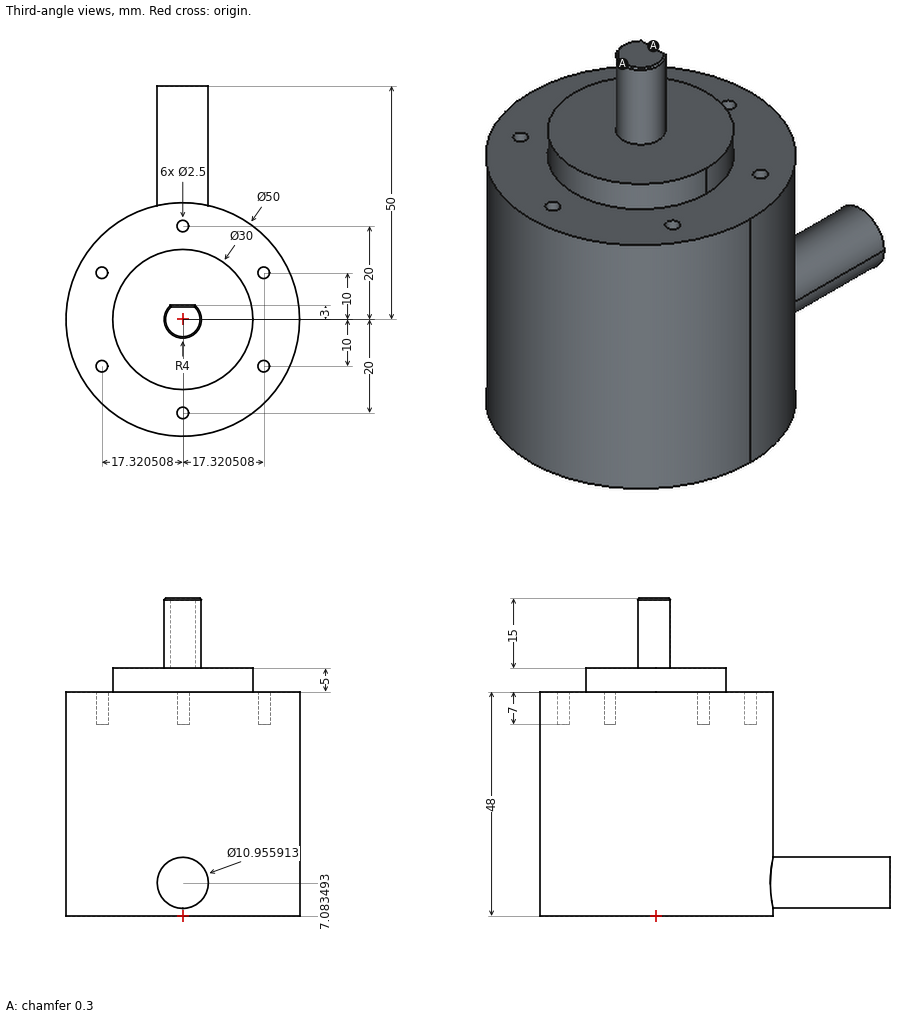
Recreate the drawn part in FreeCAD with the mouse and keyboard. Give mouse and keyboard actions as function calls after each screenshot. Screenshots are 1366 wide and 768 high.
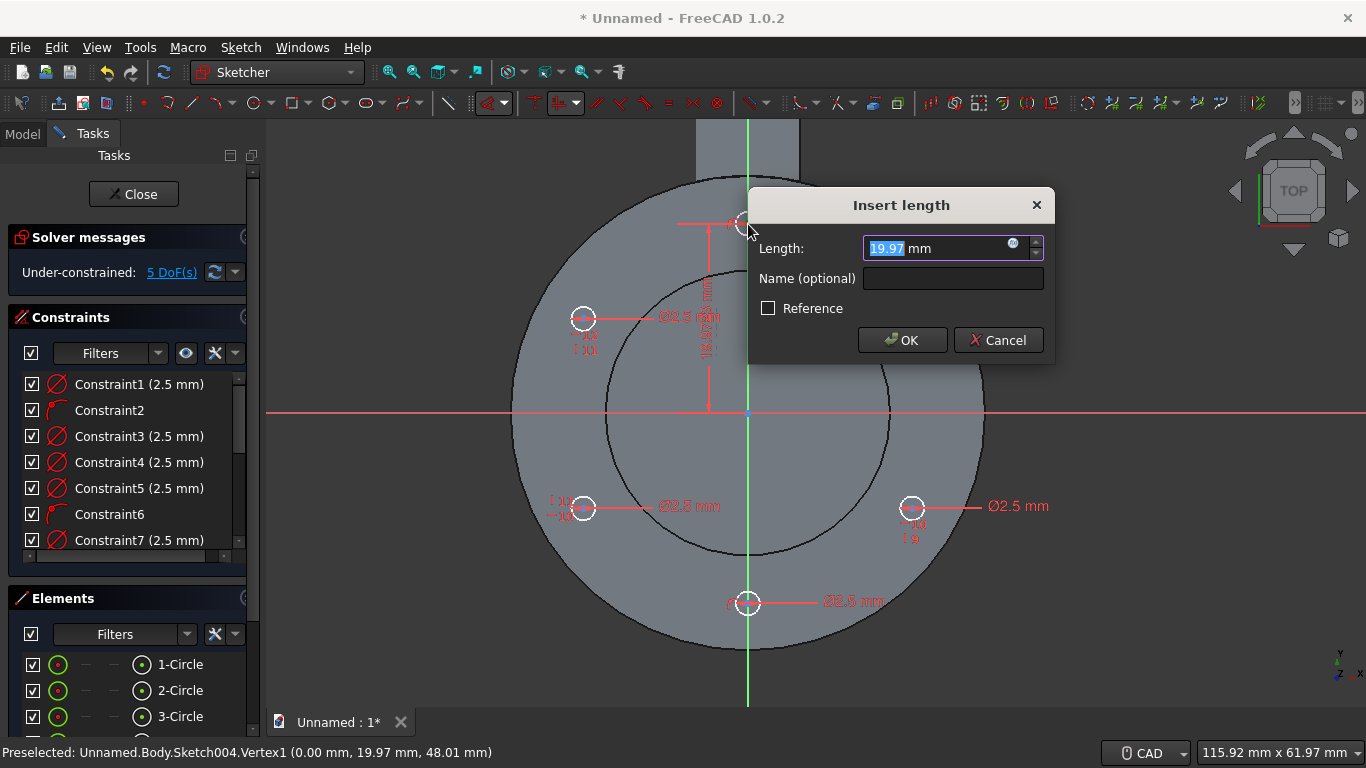
text(20)
key(Return)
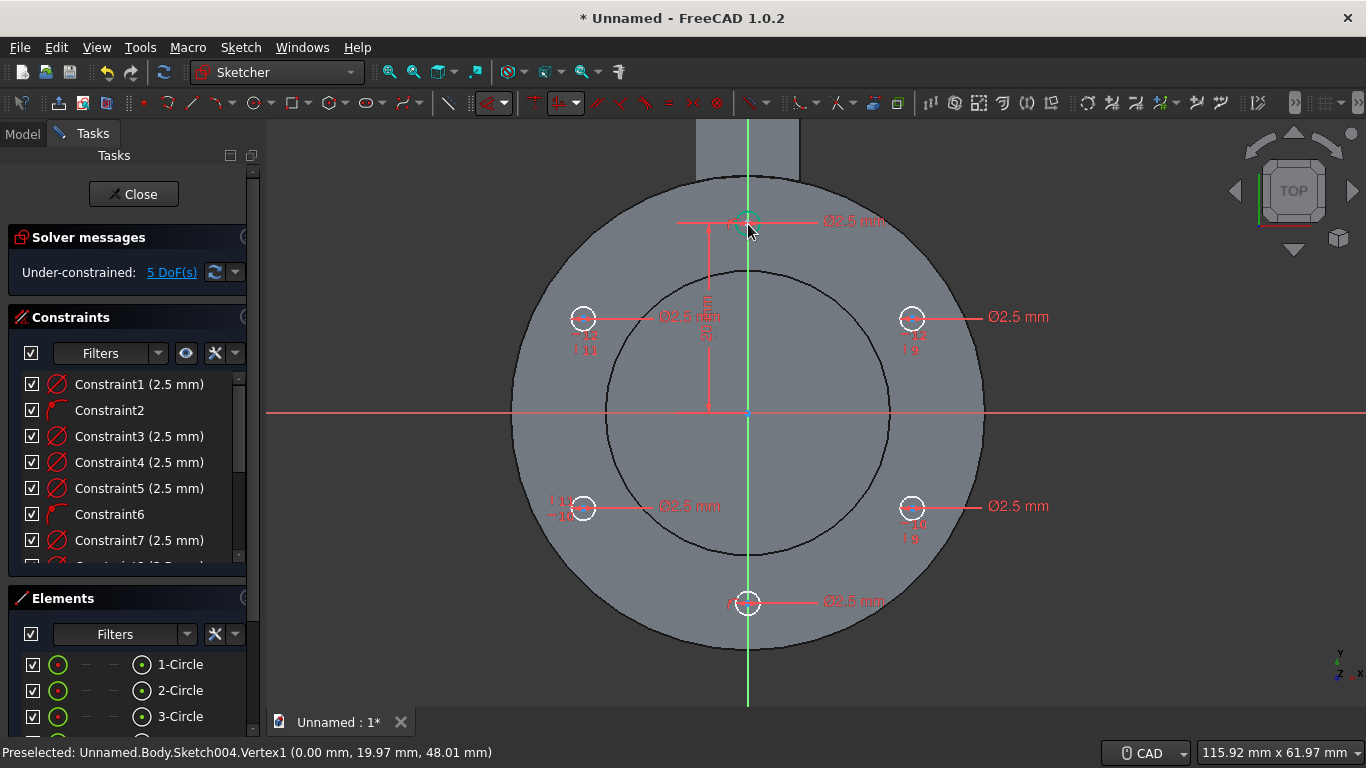
click(912, 319)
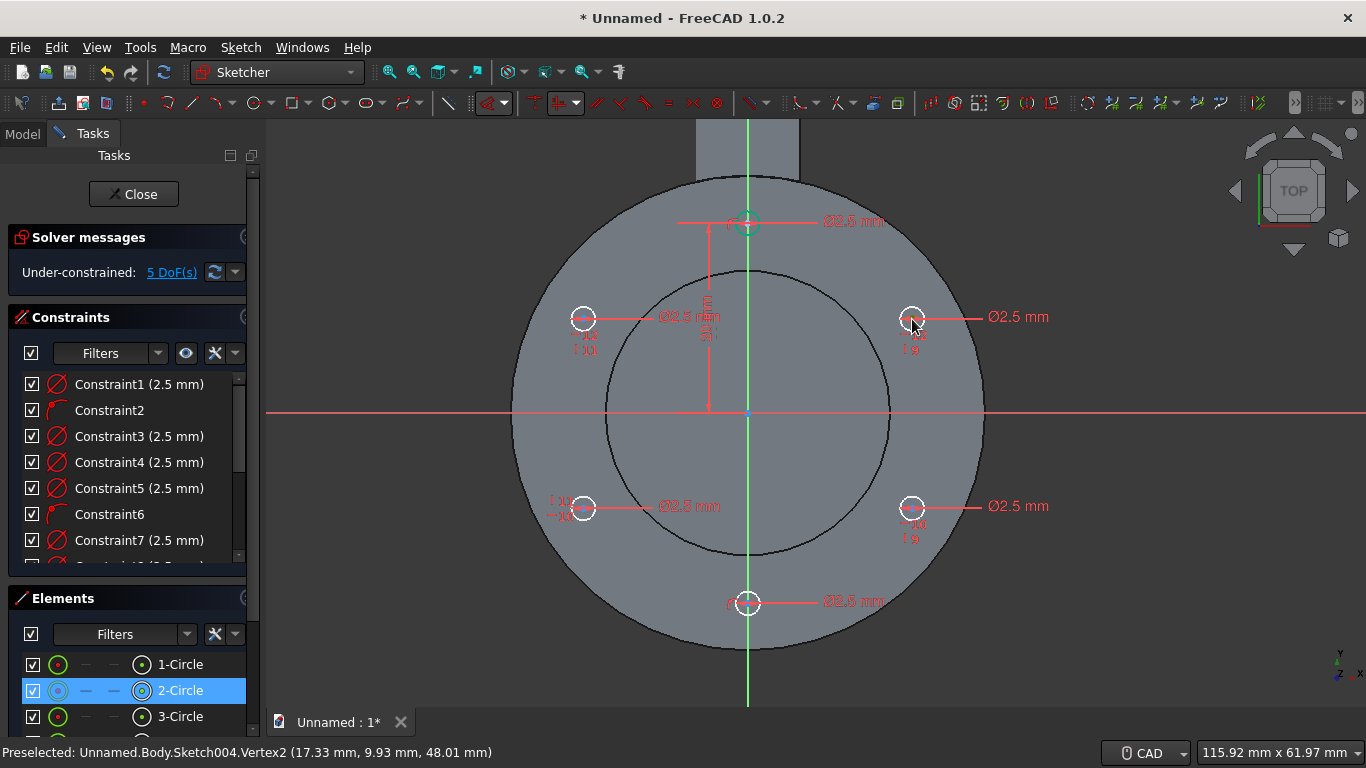
key(i)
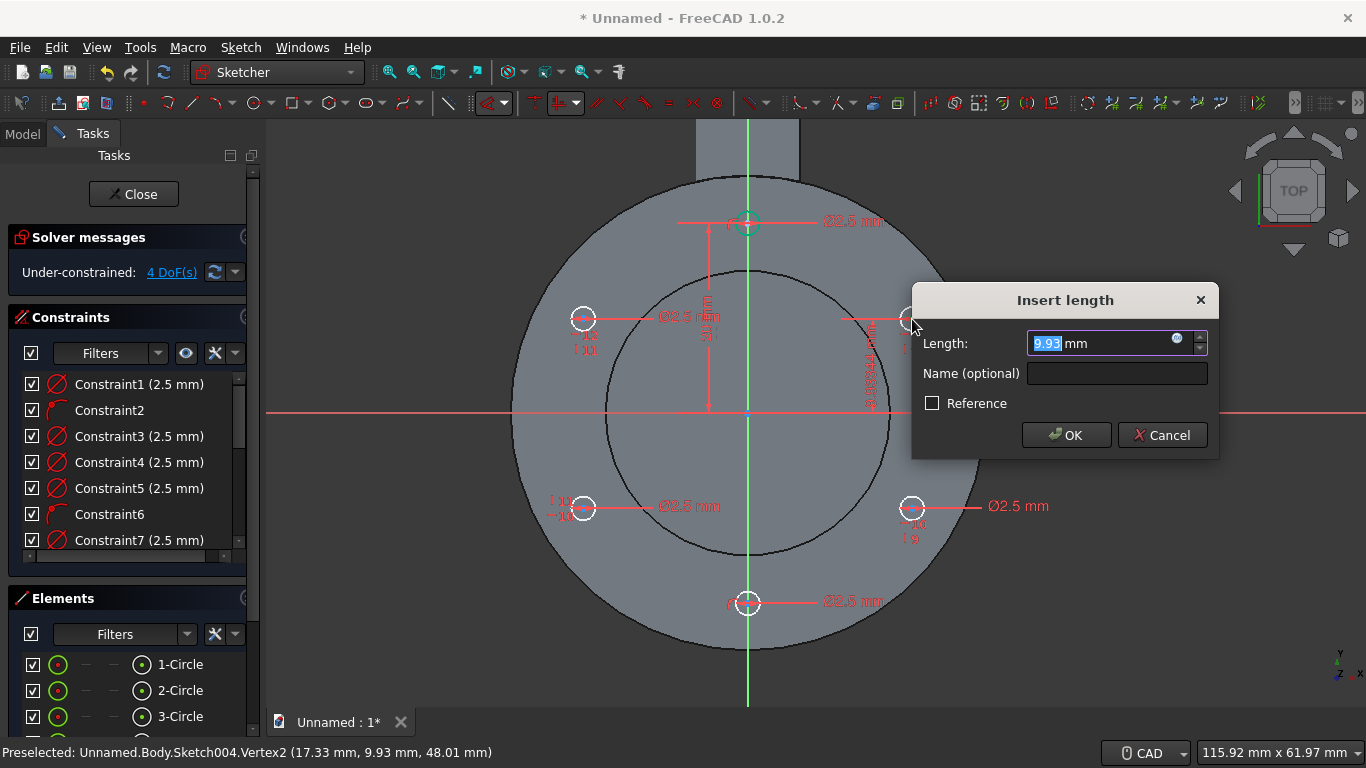
text(10)
key(Return)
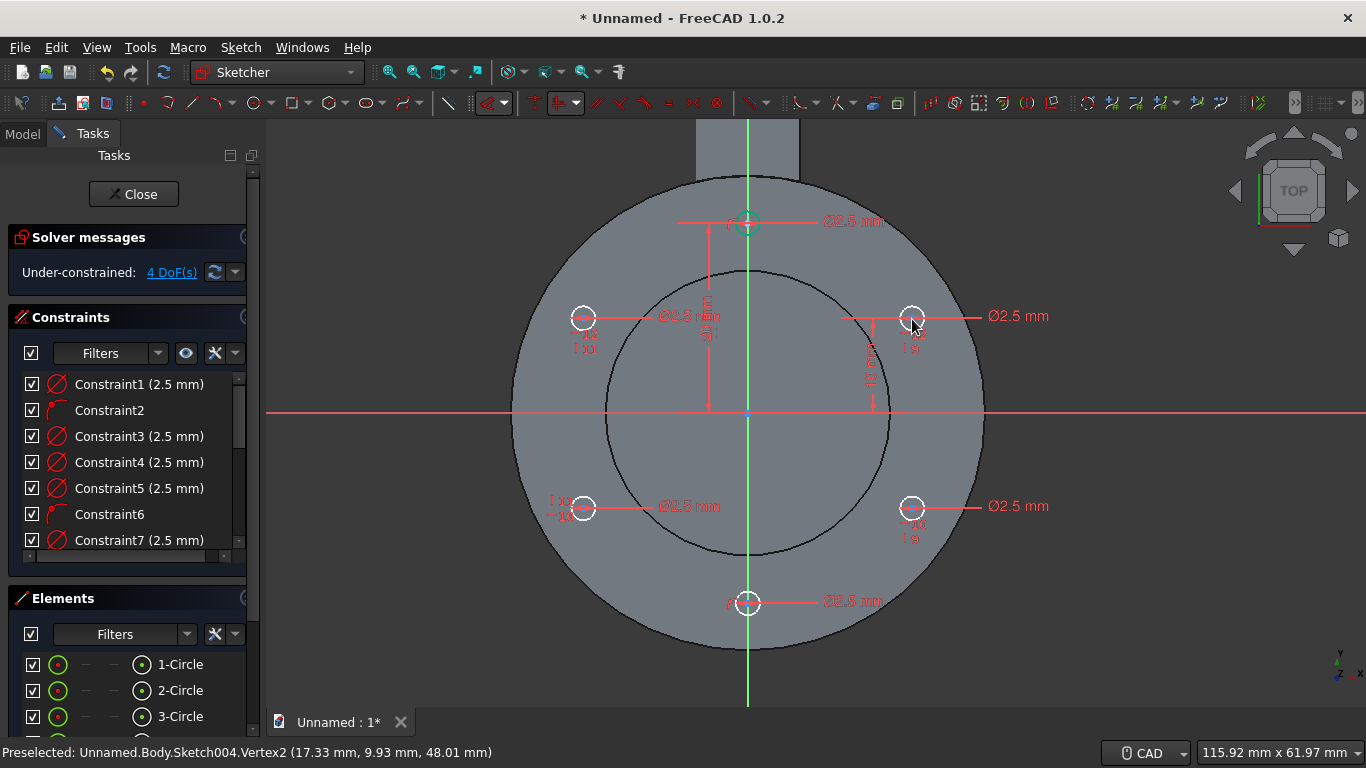
click(912, 508)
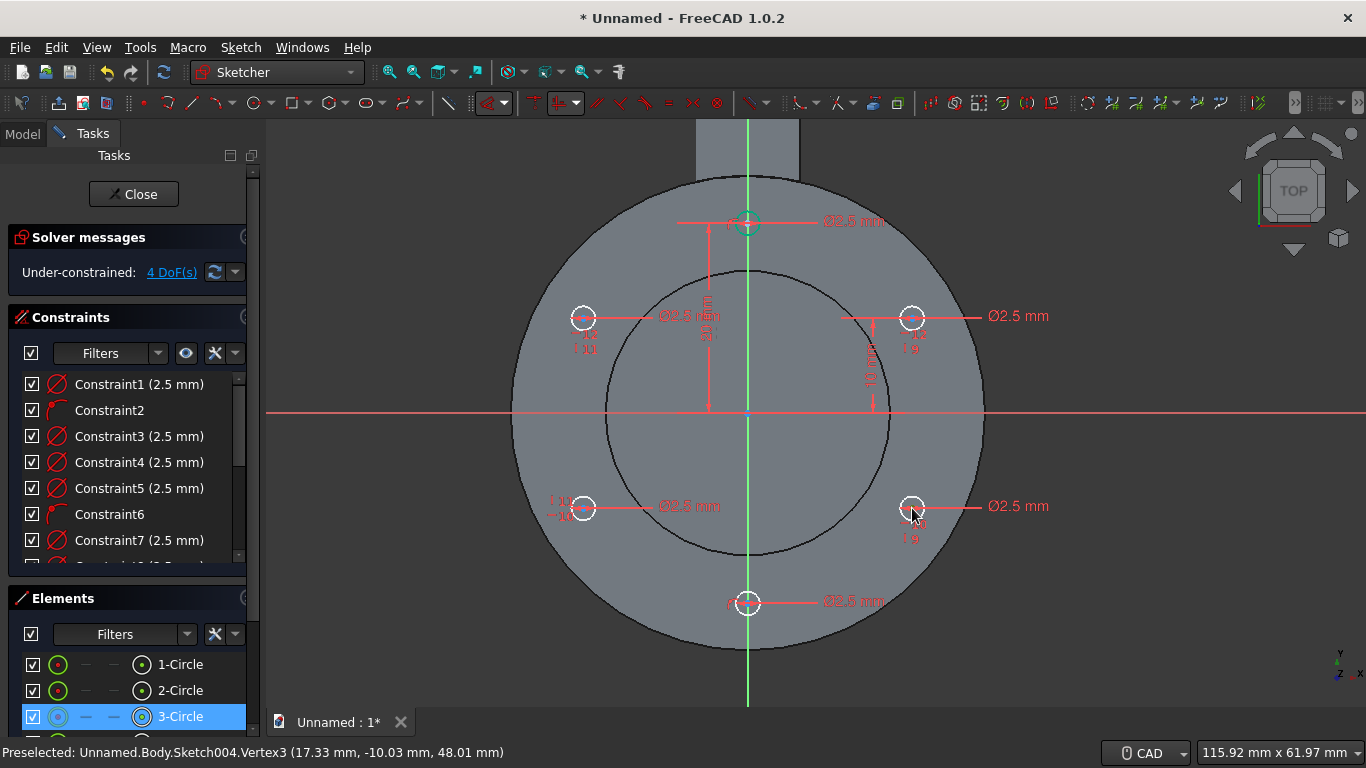
click(506, 104)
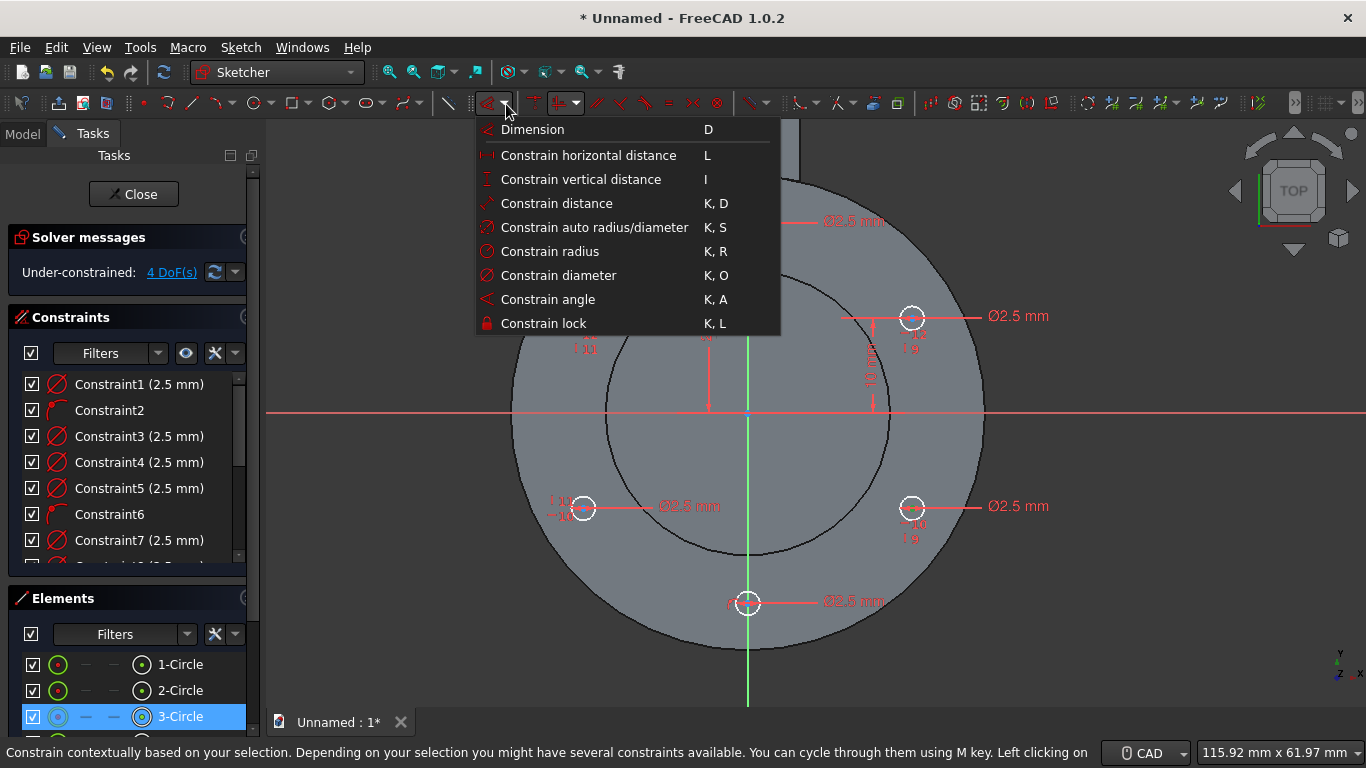
click(628, 179)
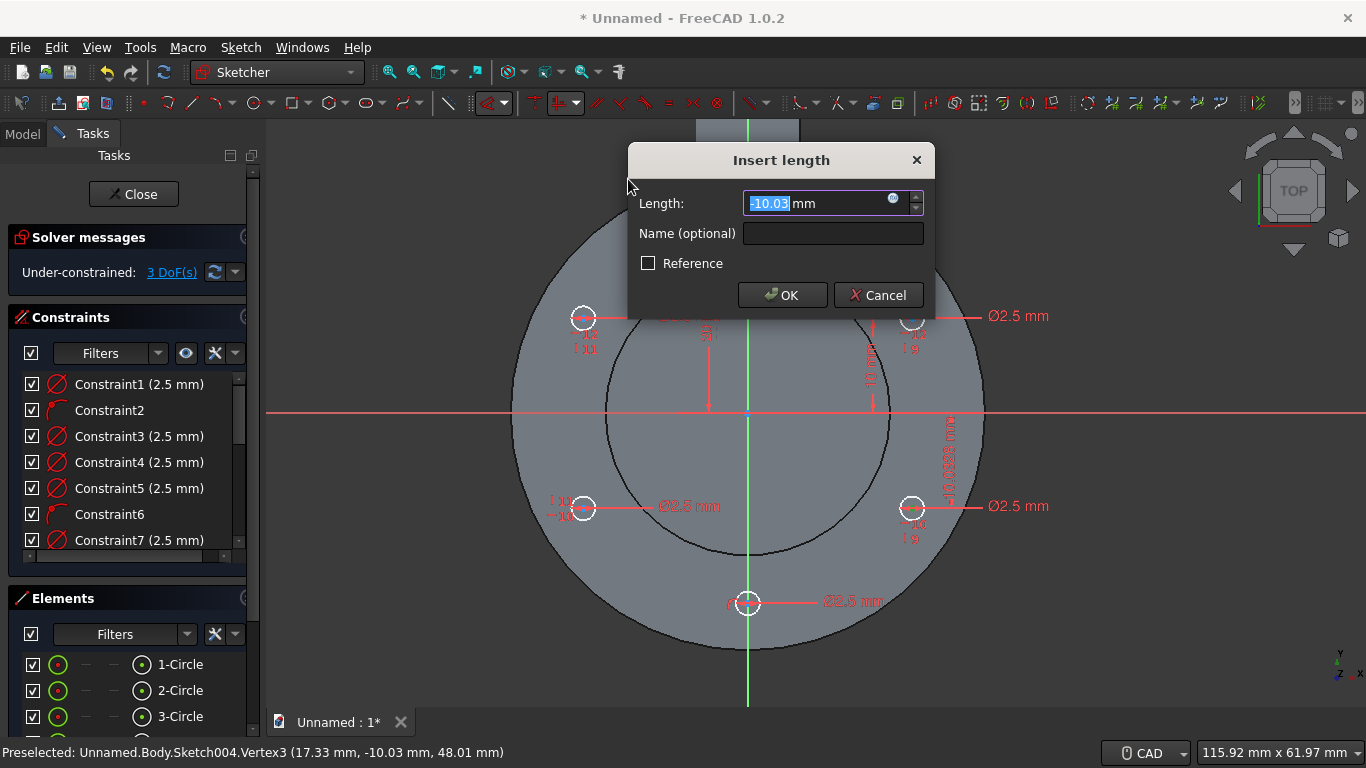
text(-10)
key(Return)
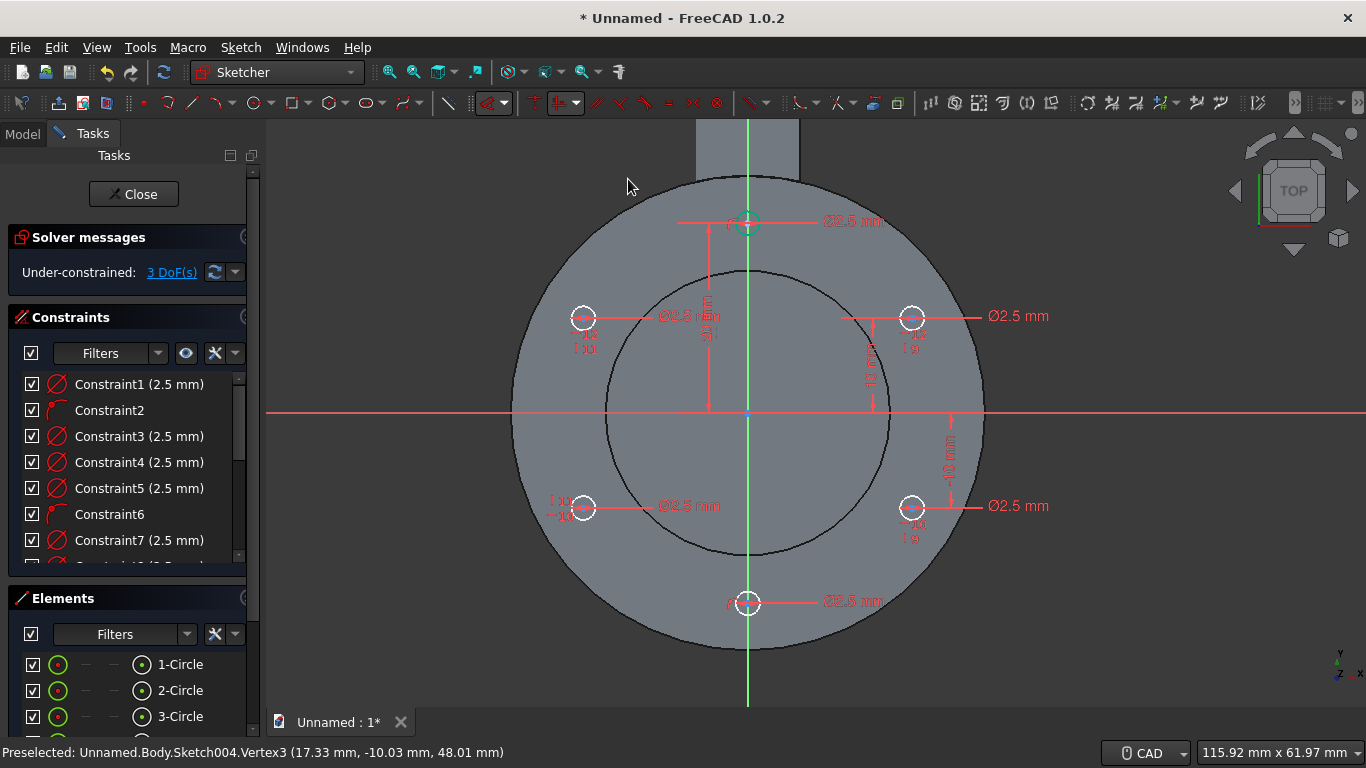
click(748, 603)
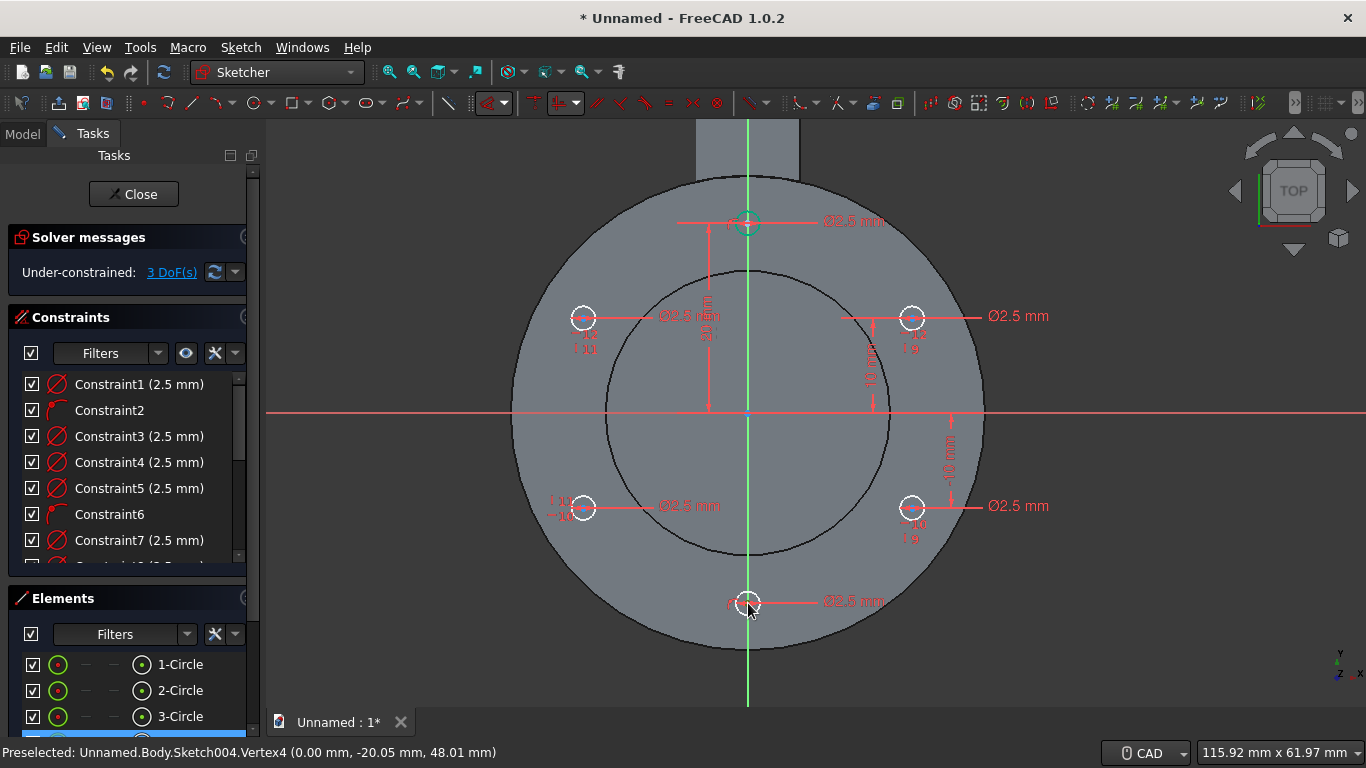
click(506, 104)